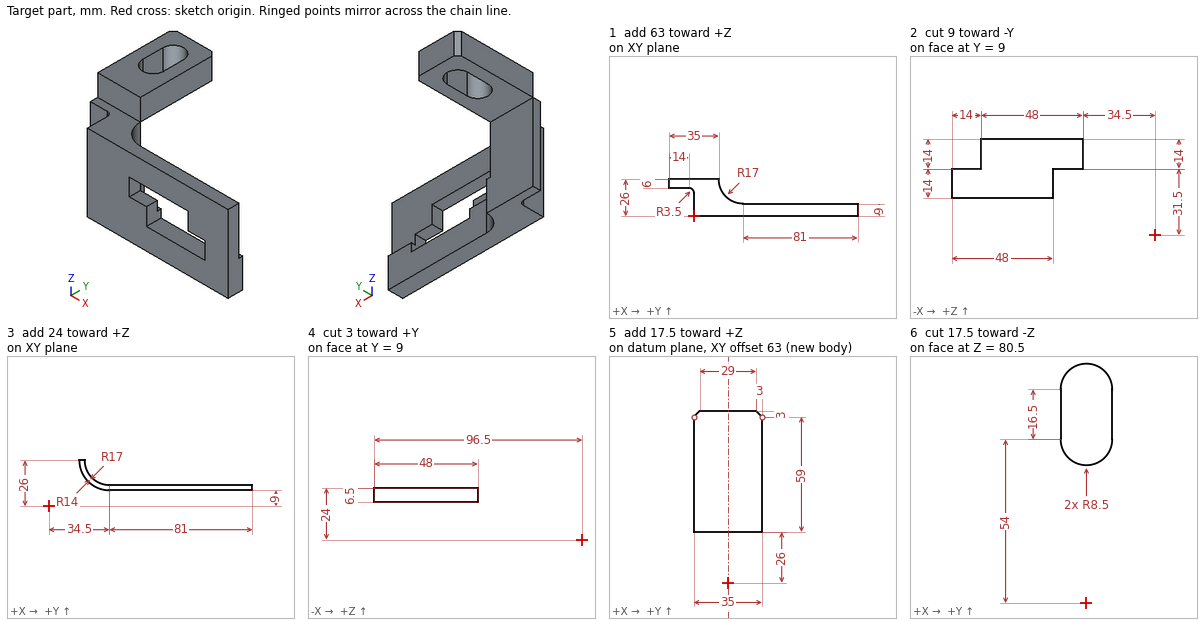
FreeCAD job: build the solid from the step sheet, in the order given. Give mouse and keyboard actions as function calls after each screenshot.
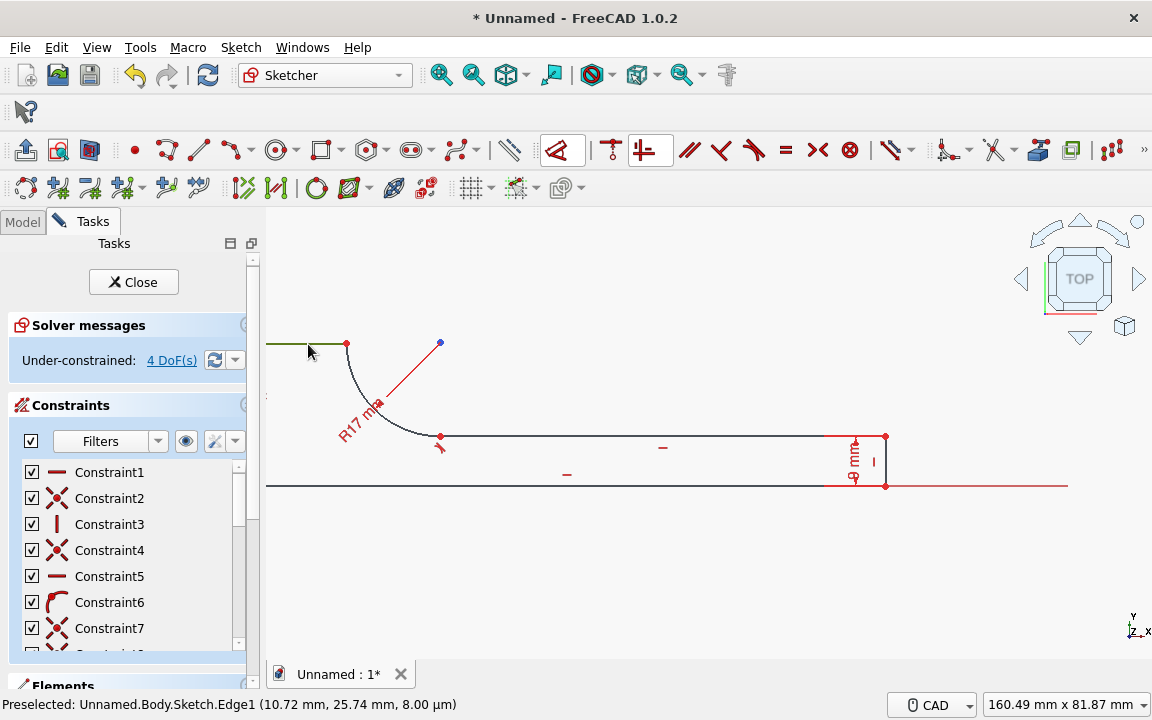
click(580, 150)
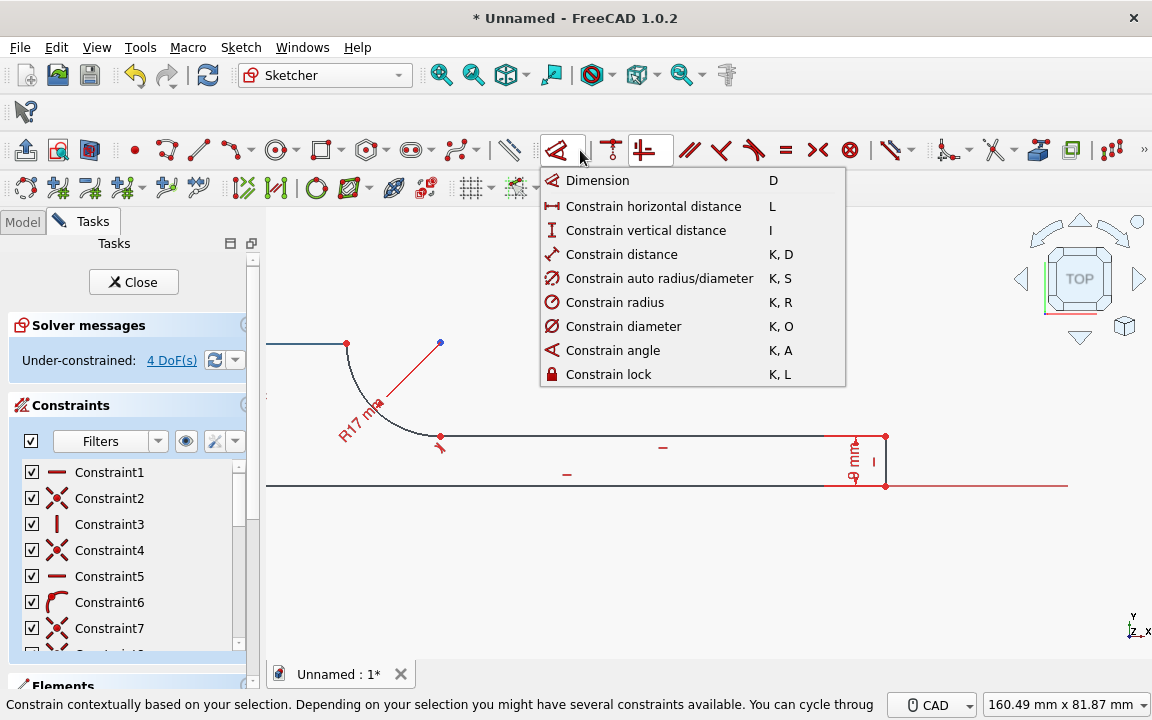
click(693, 206)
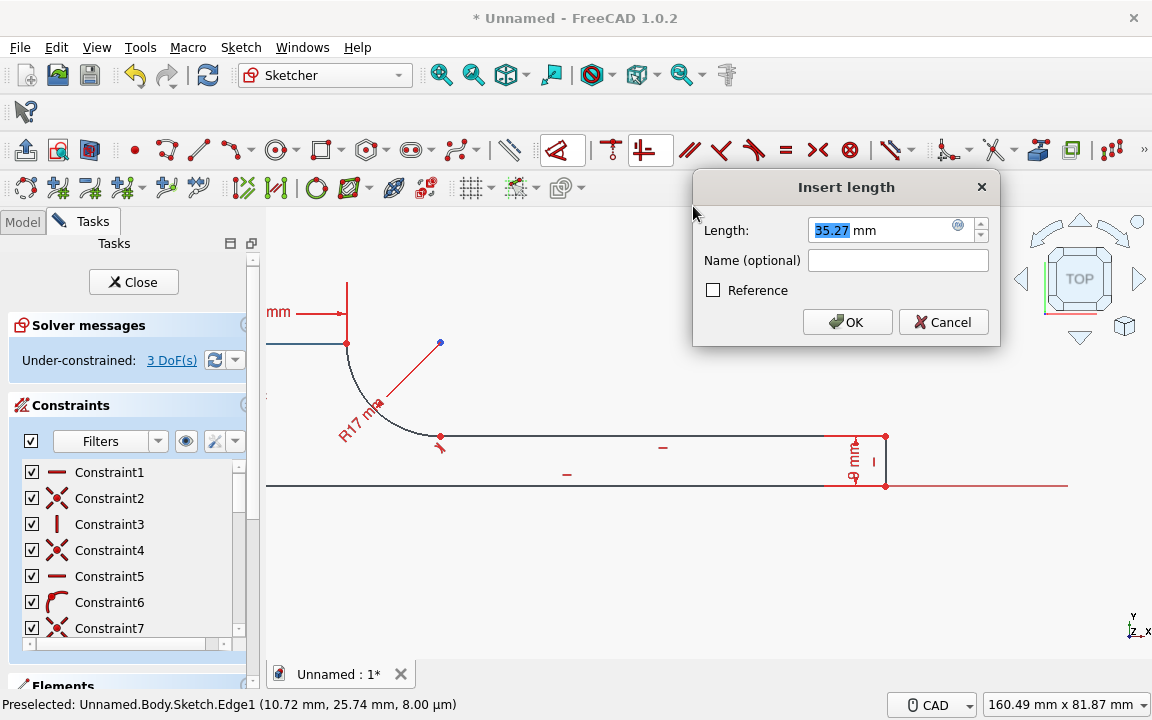
text(35)
key(Return)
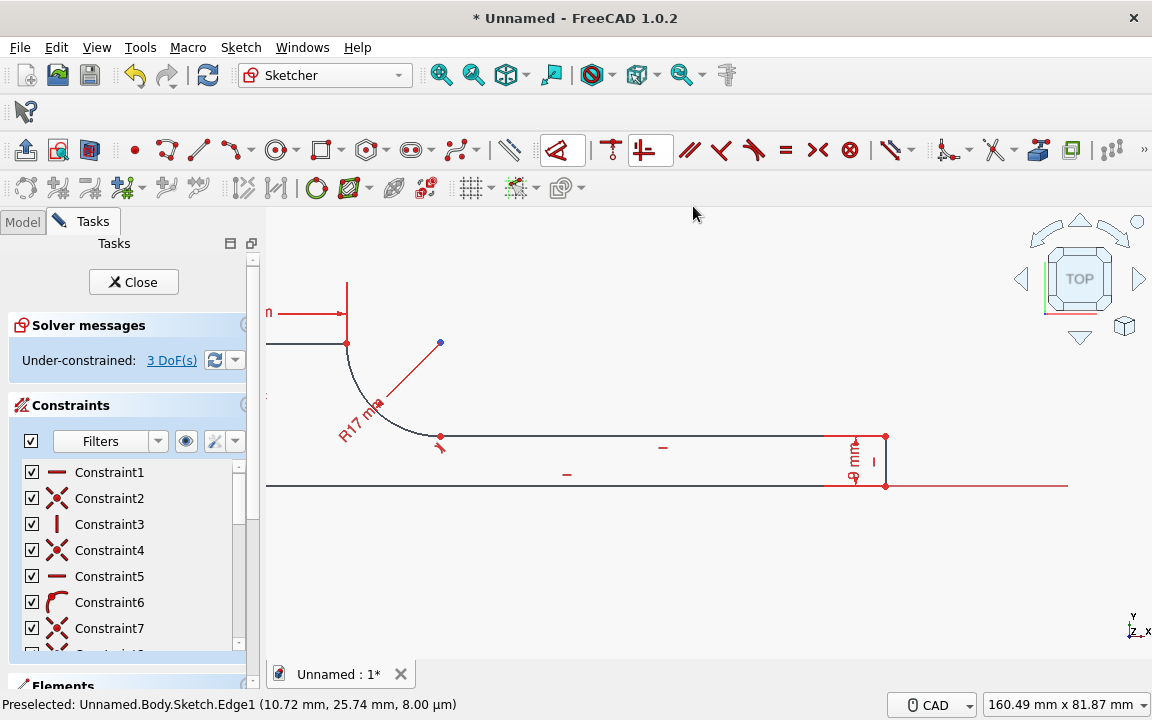
scroll(887, 471, down, 2)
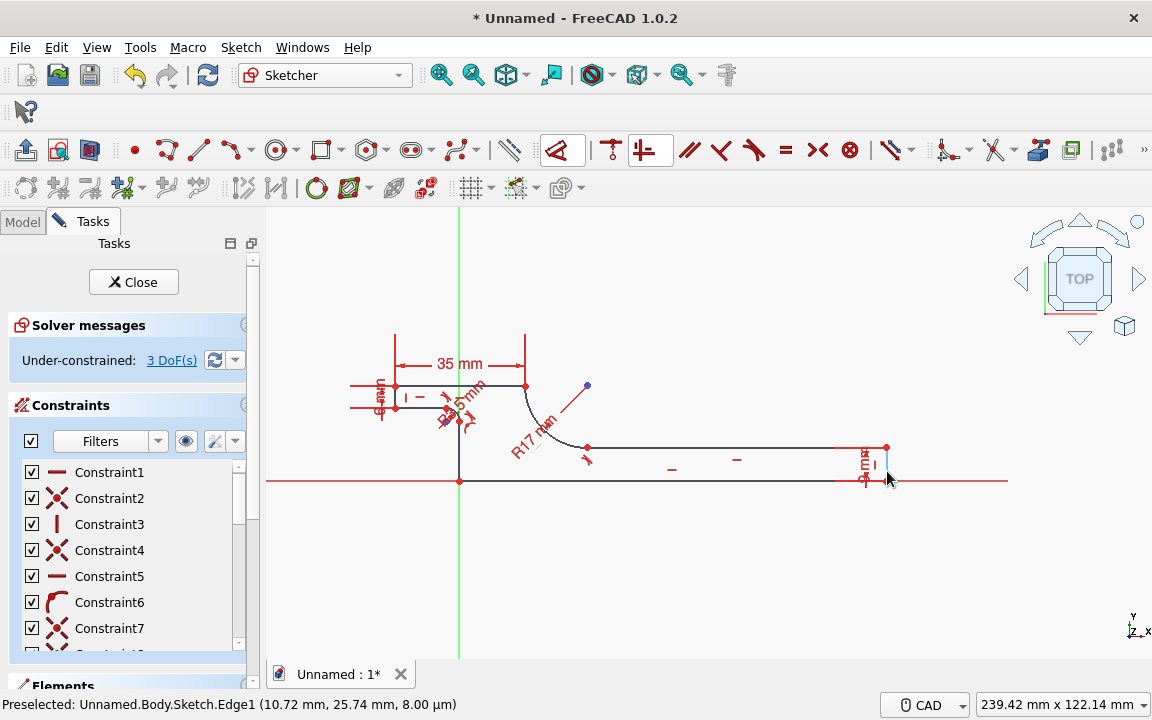
click(411, 408)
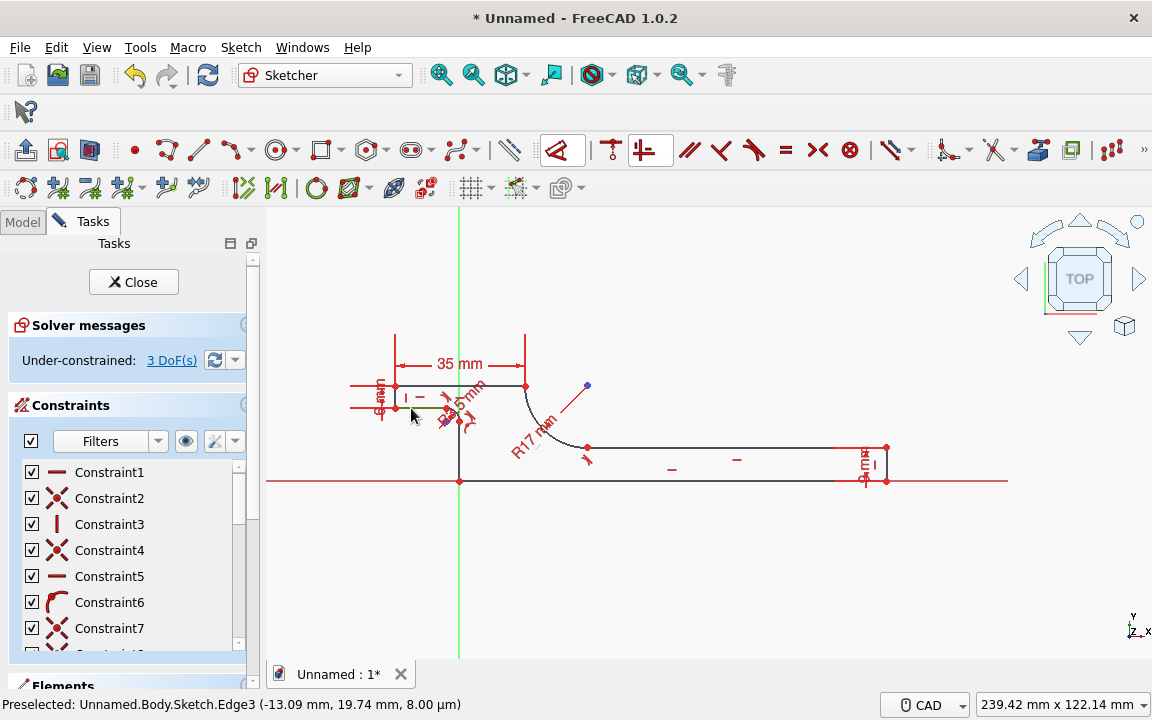
key(l)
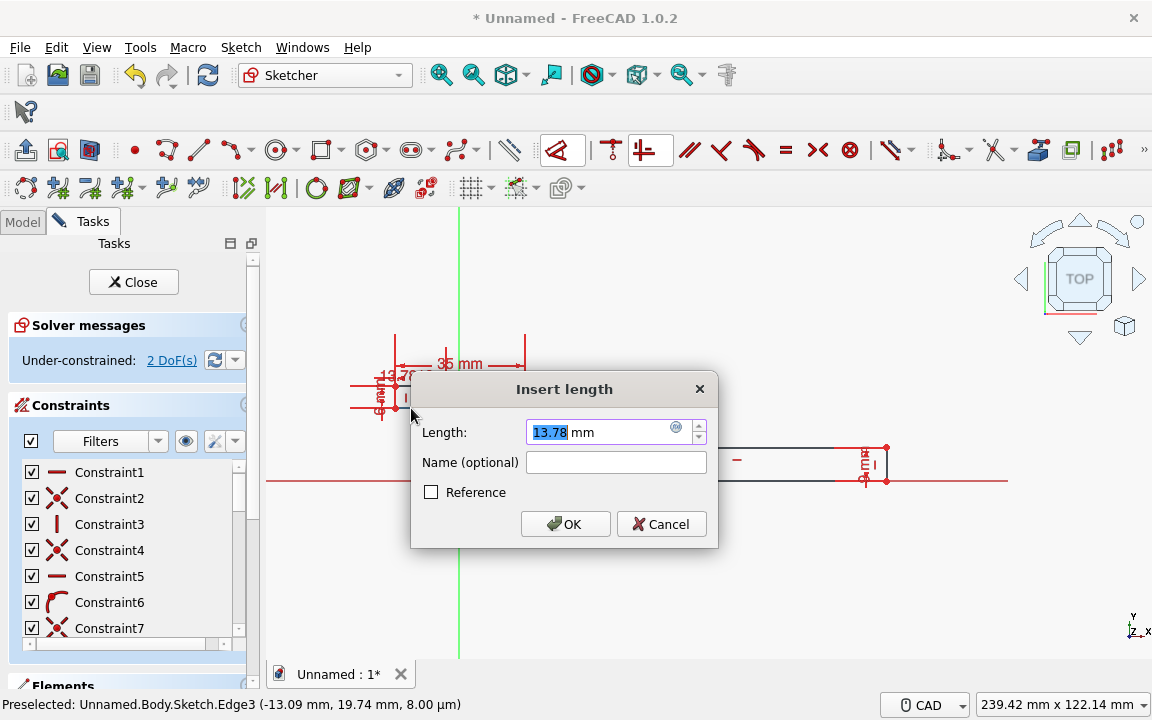
text(14)
key(Return)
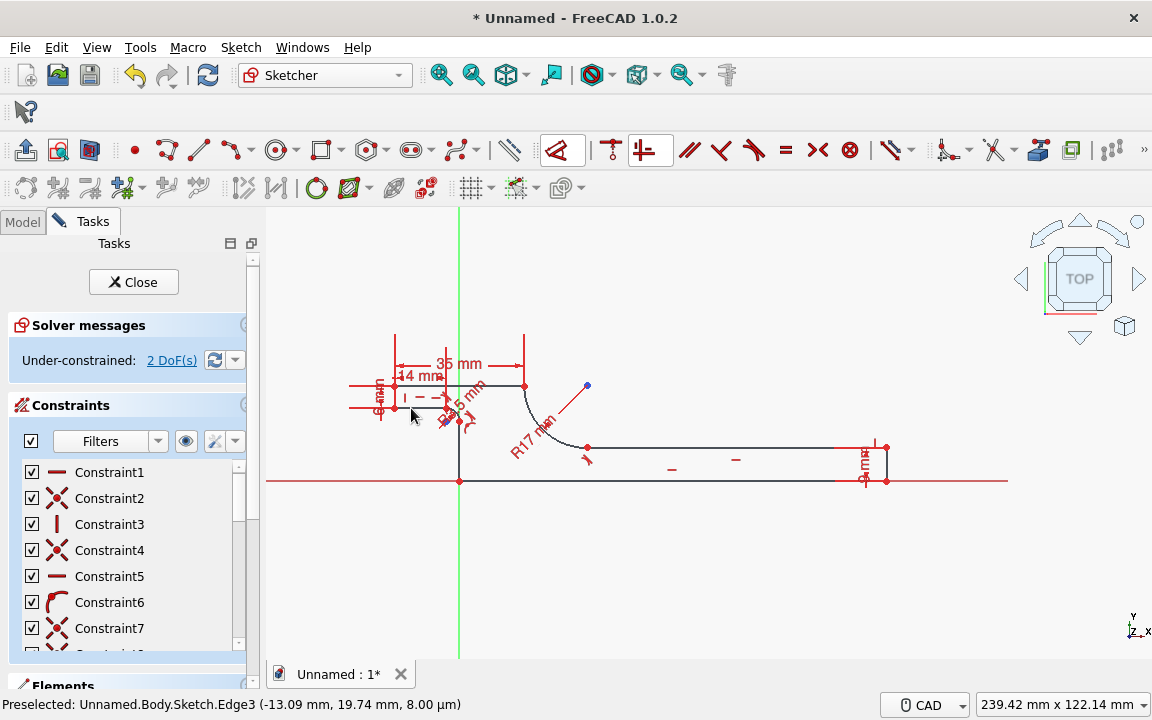
click(797, 448)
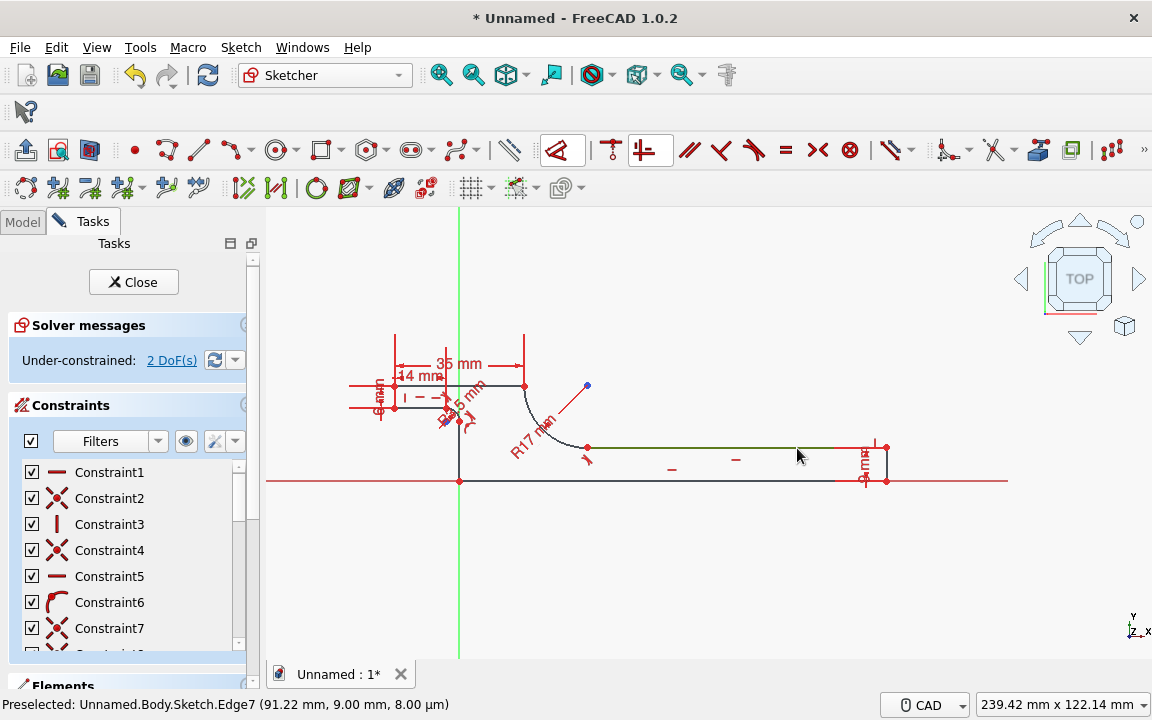
key(l)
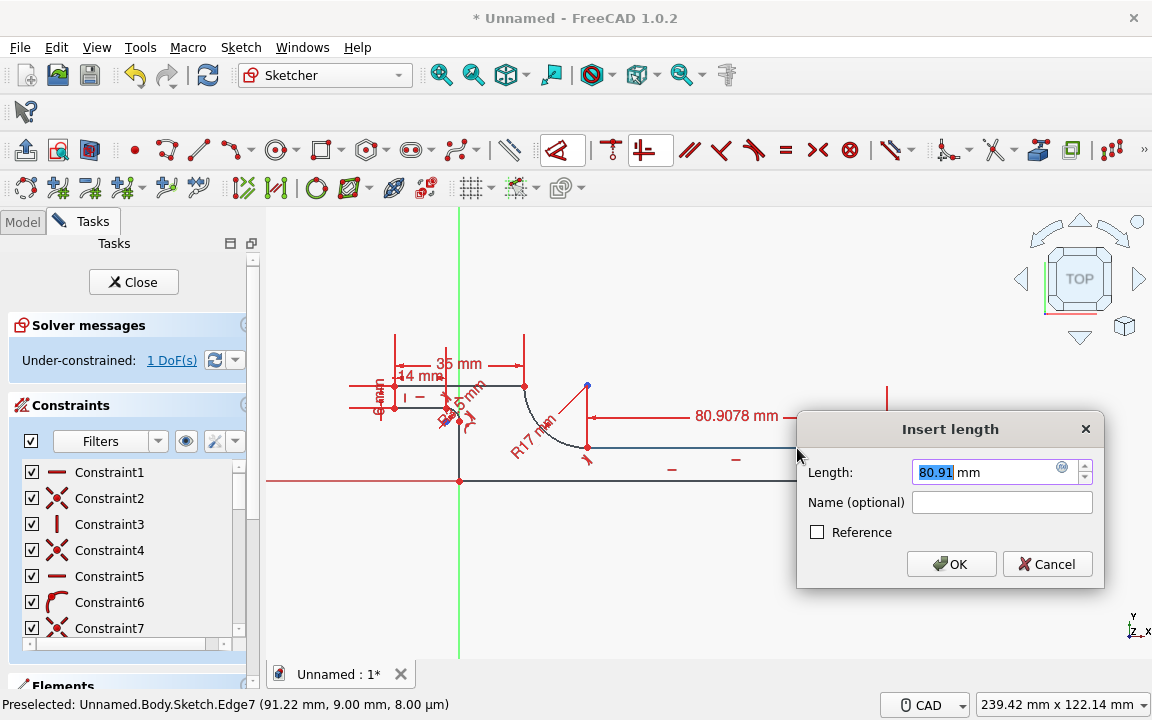
text(81)
key(Return)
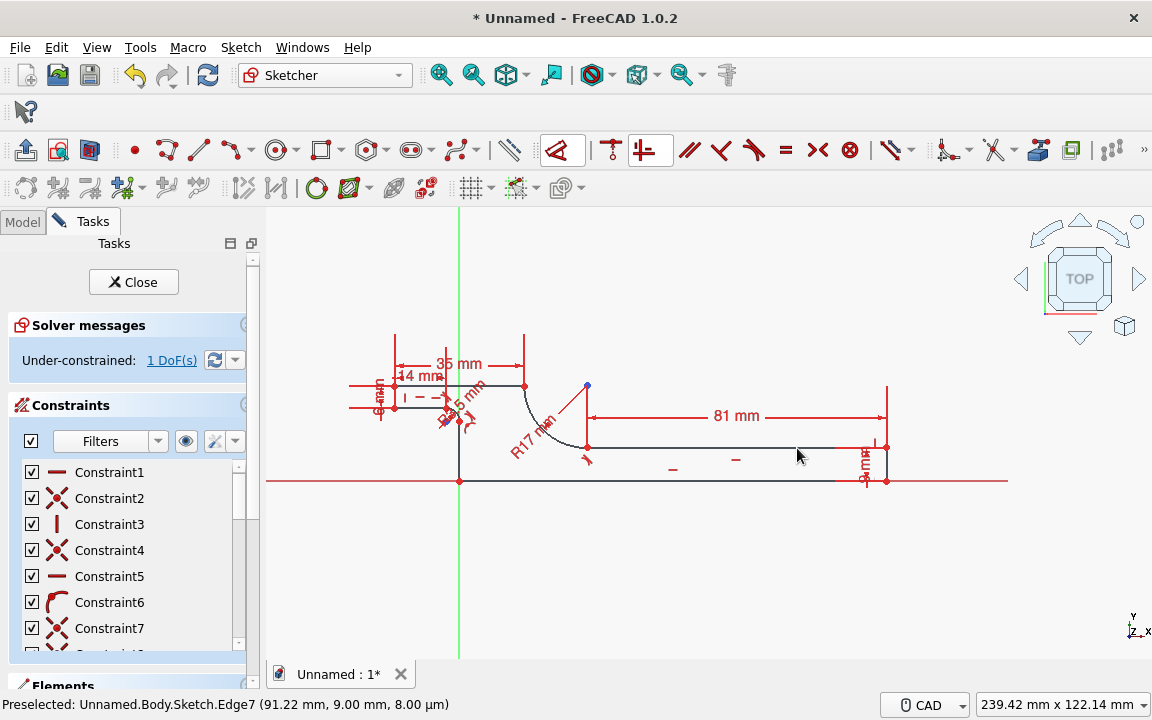
click(524, 386)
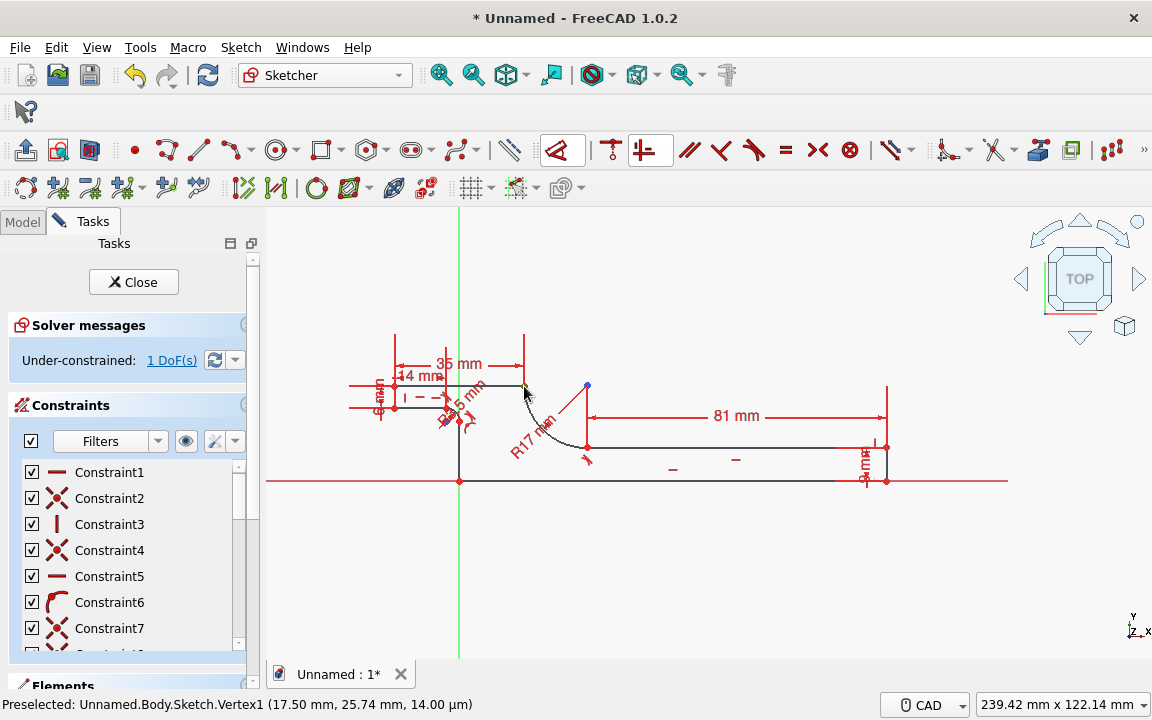
key(i)